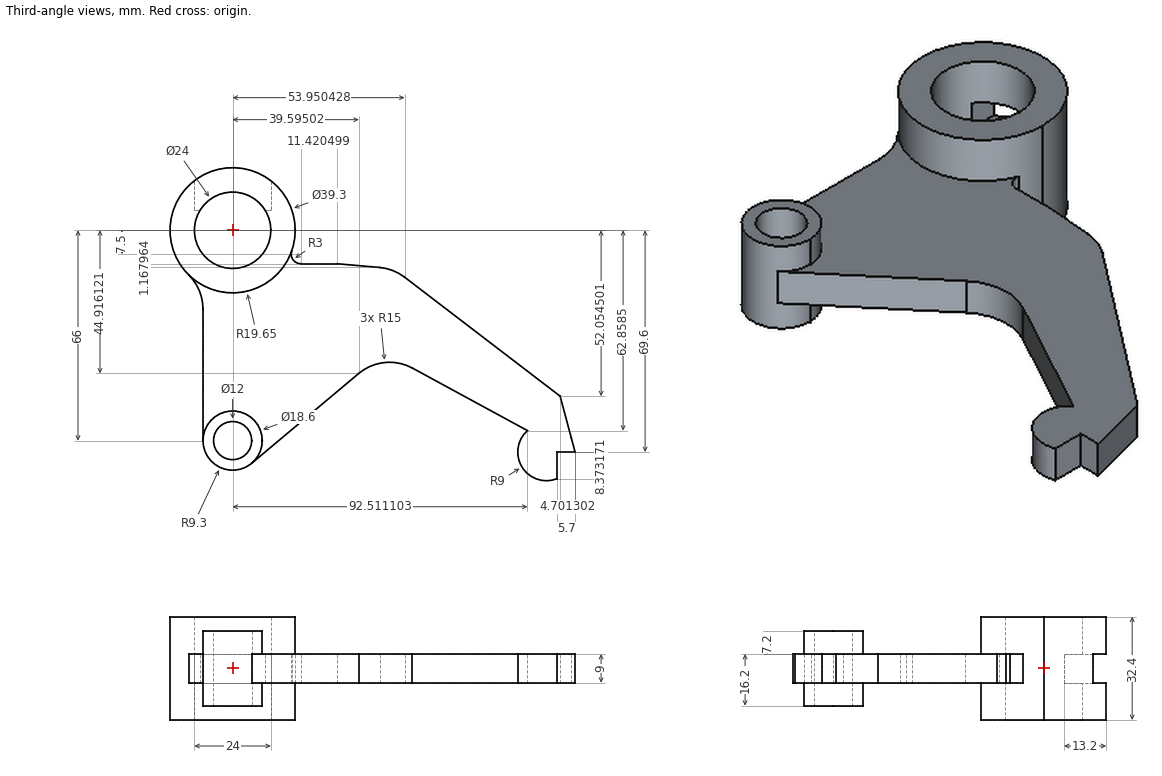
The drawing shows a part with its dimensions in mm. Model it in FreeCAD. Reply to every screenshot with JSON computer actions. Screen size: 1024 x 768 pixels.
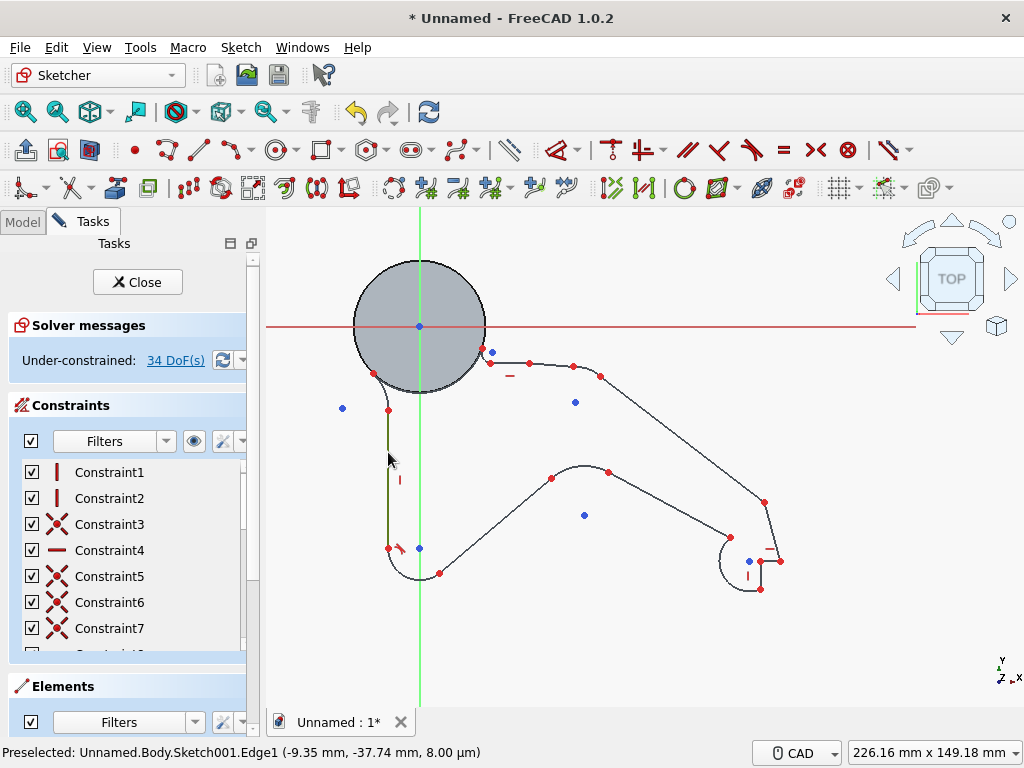
{"action": "left_click", "coordinate": [387, 399]}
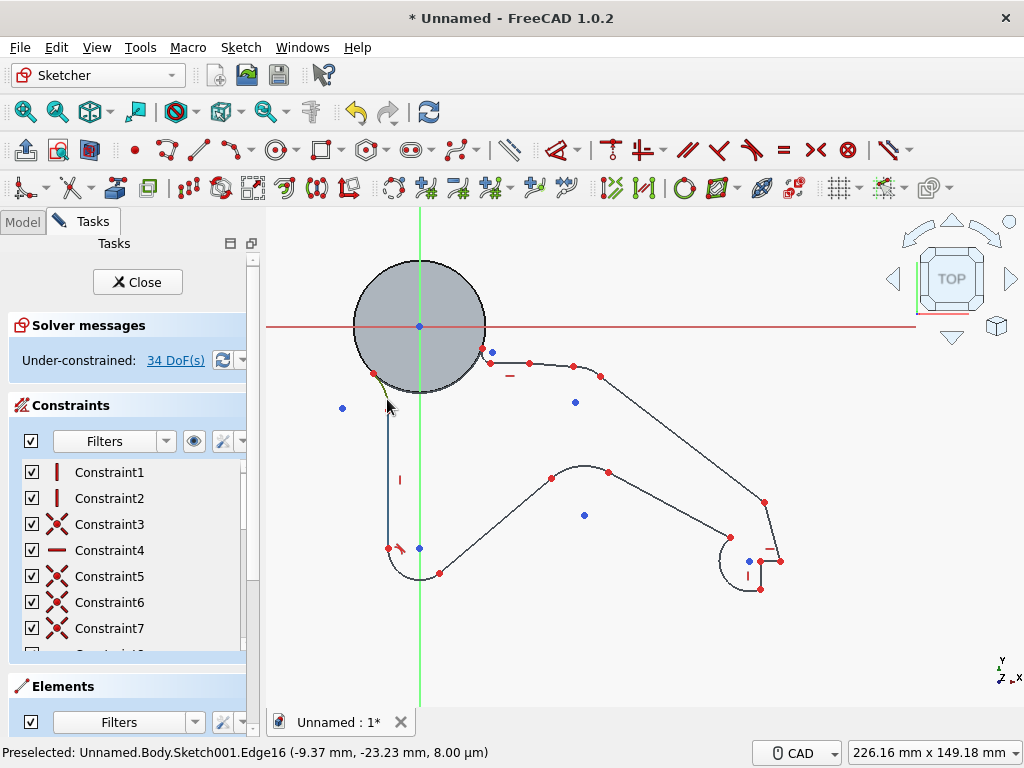
{"action": "key", "text": "t"}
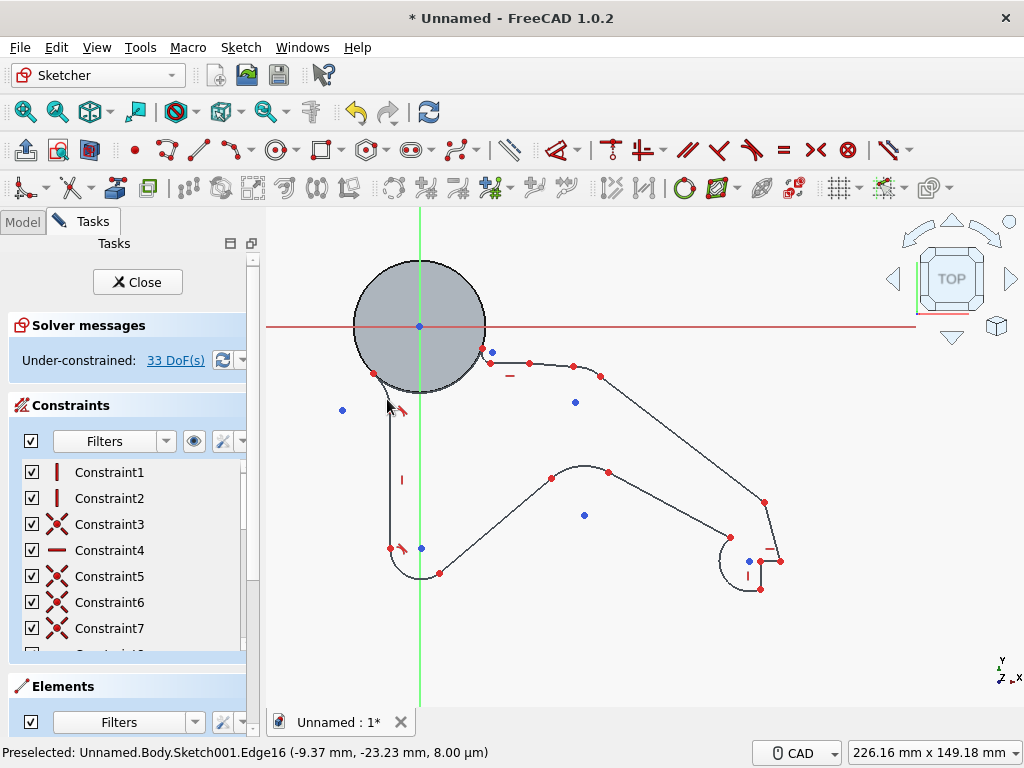
{"action": "left_click", "coordinate": [473, 545]}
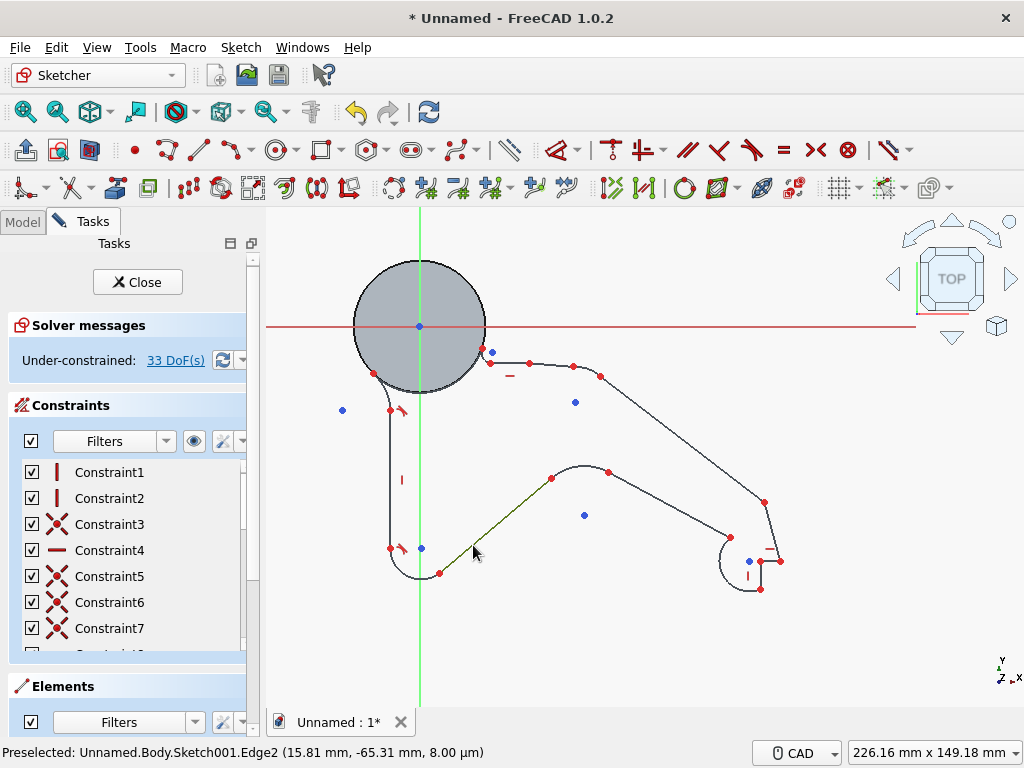
{"action": "left_click", "coordinate": [397, 567]}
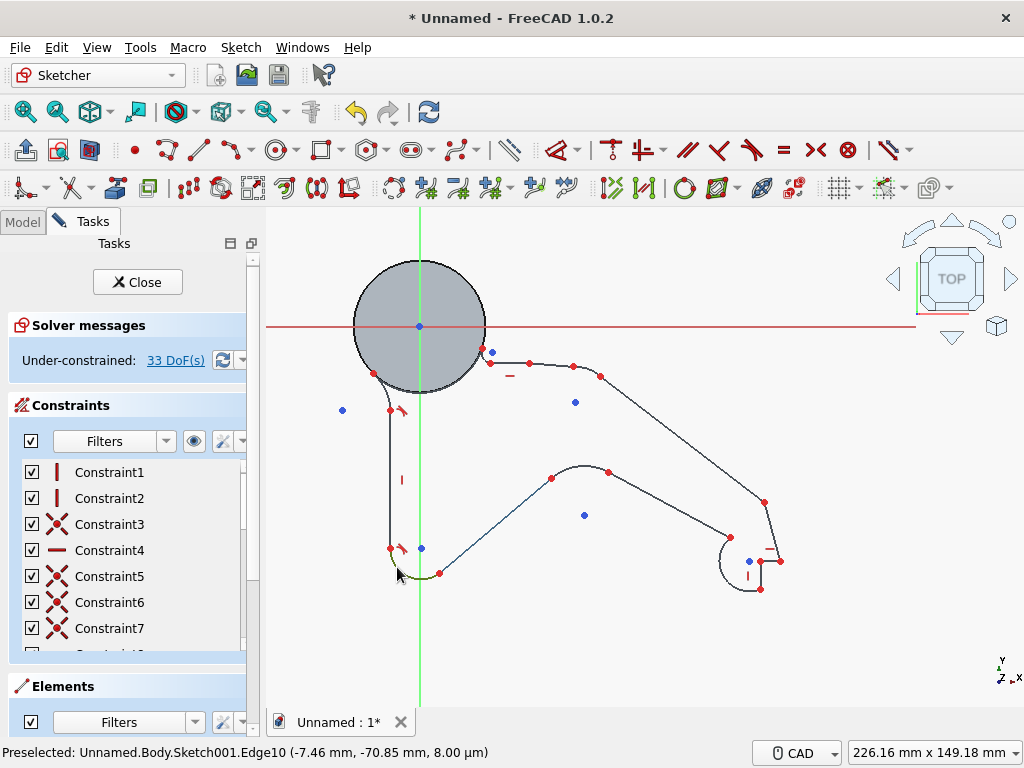
{"action": "key", "text": "t"}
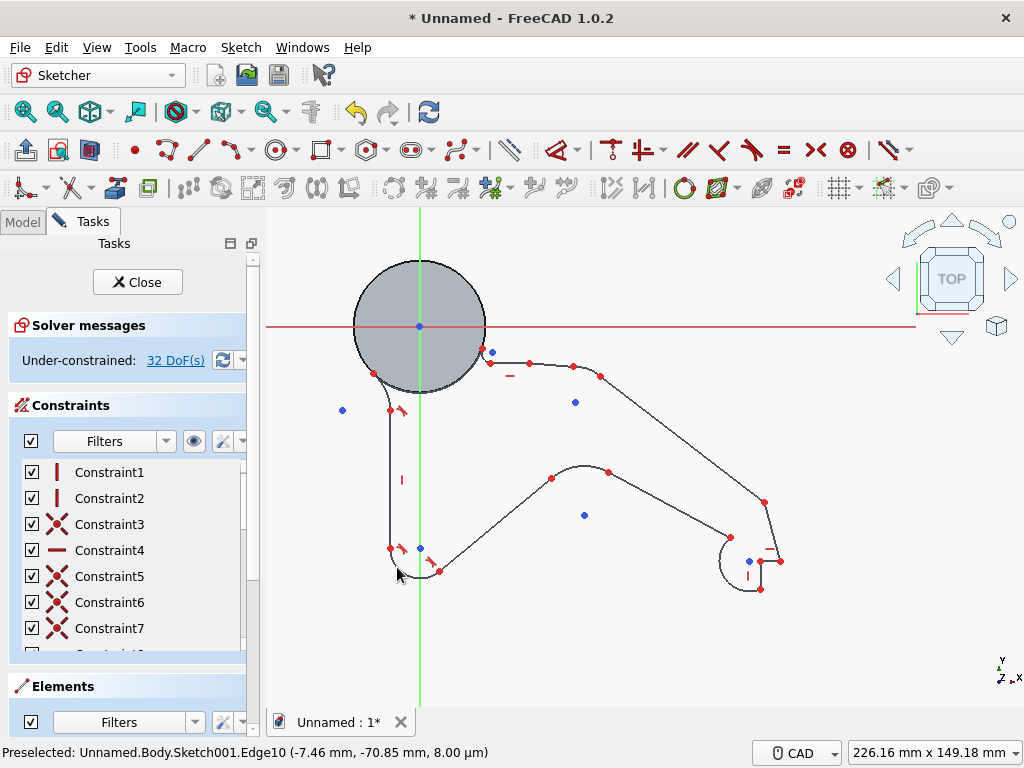
{"action": "left_click", "coordinate": [473, 543]}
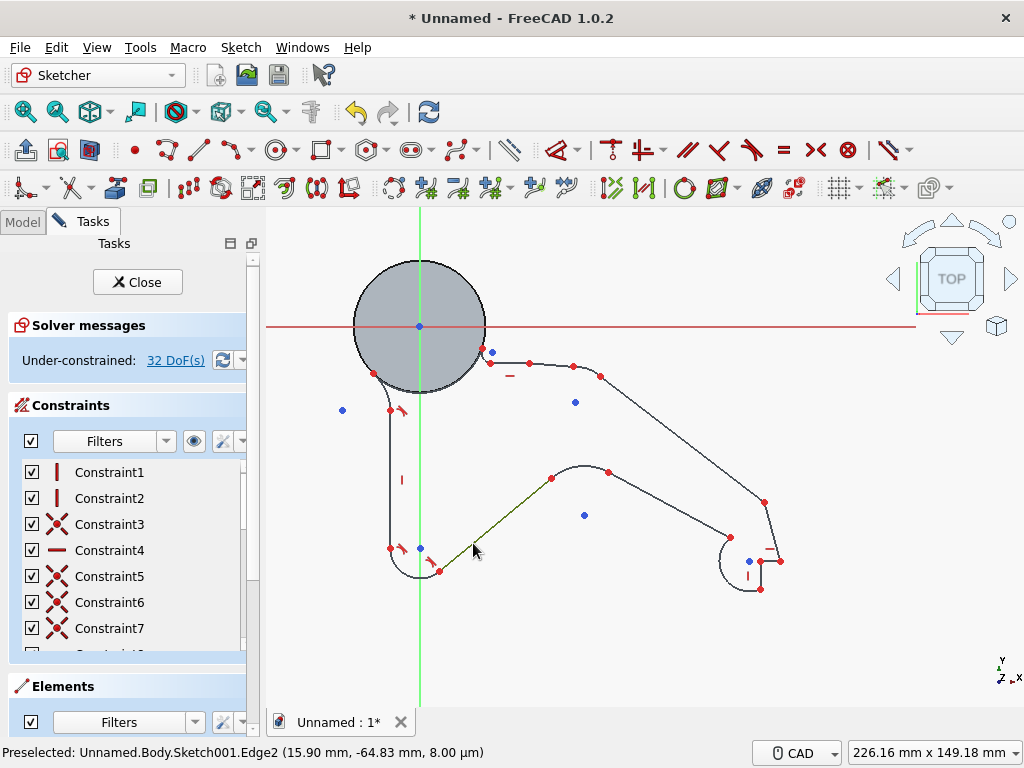
{"action": "left_click", "coordinate": [591, 466]}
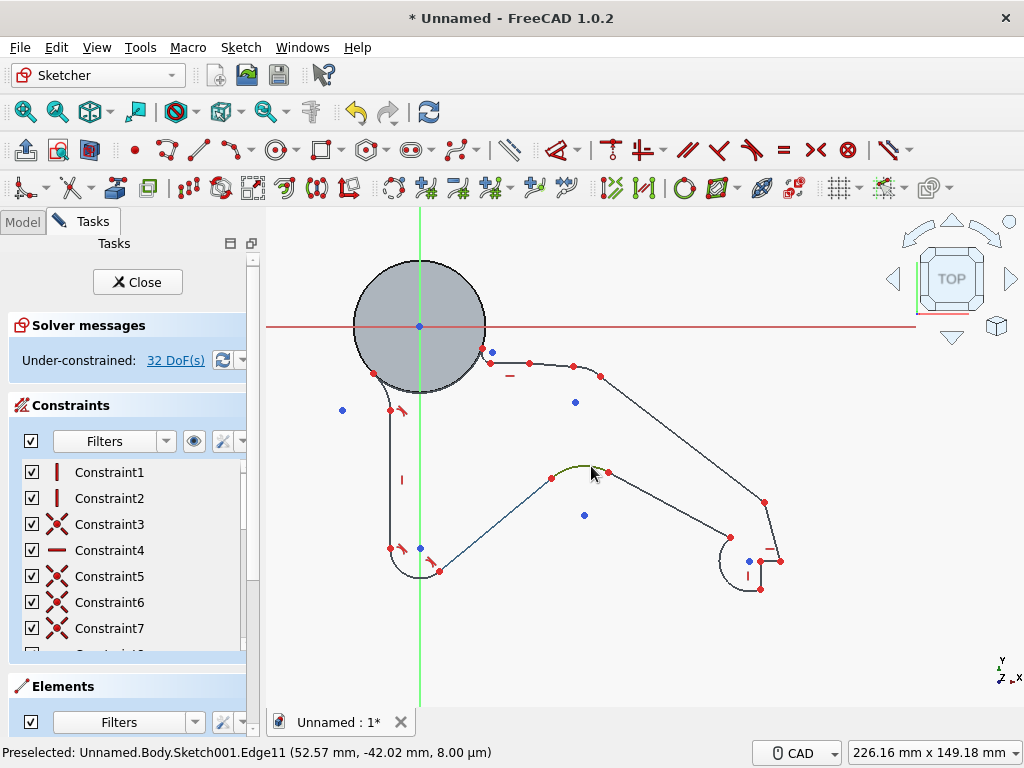
{"action": "key", "text": "t"}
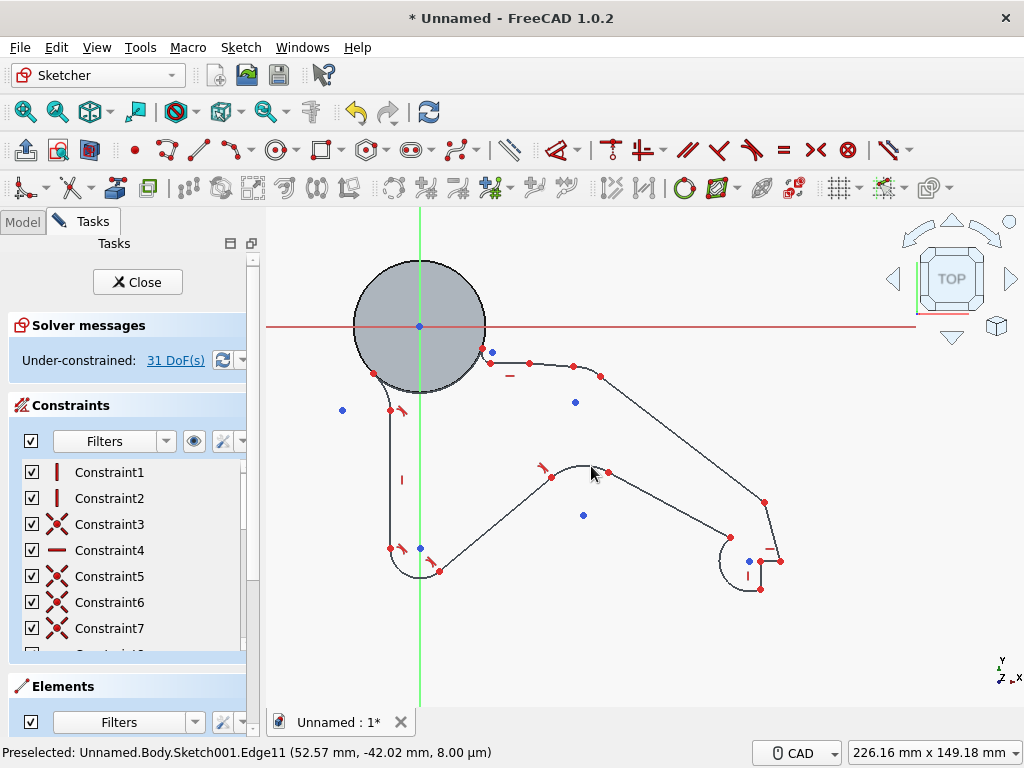
{"action": "left_click", "coordinate": [645, 492]}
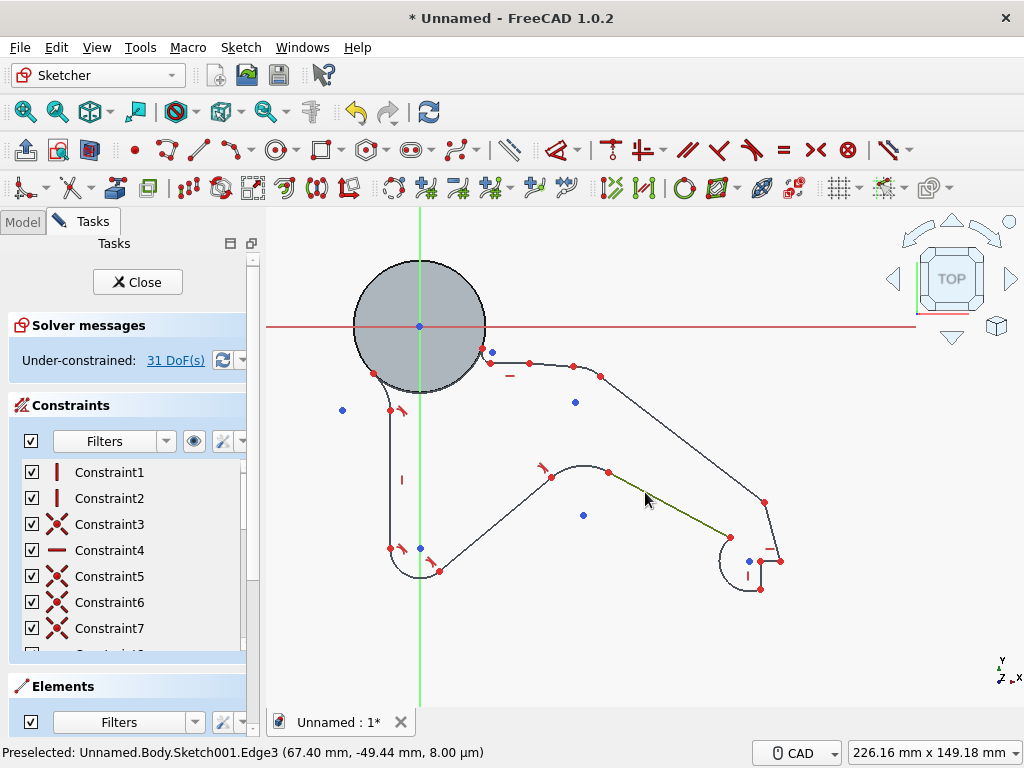
{"action": "left_click", "coordinate": [591, 466]}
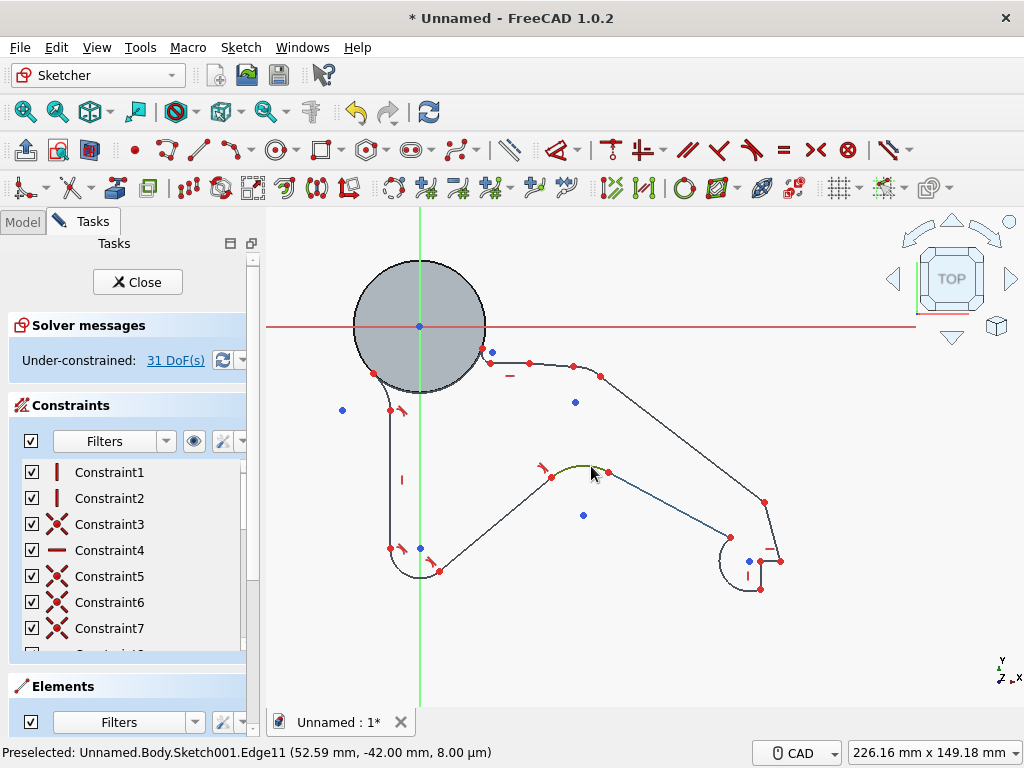
{"action": "key", "text": "t"}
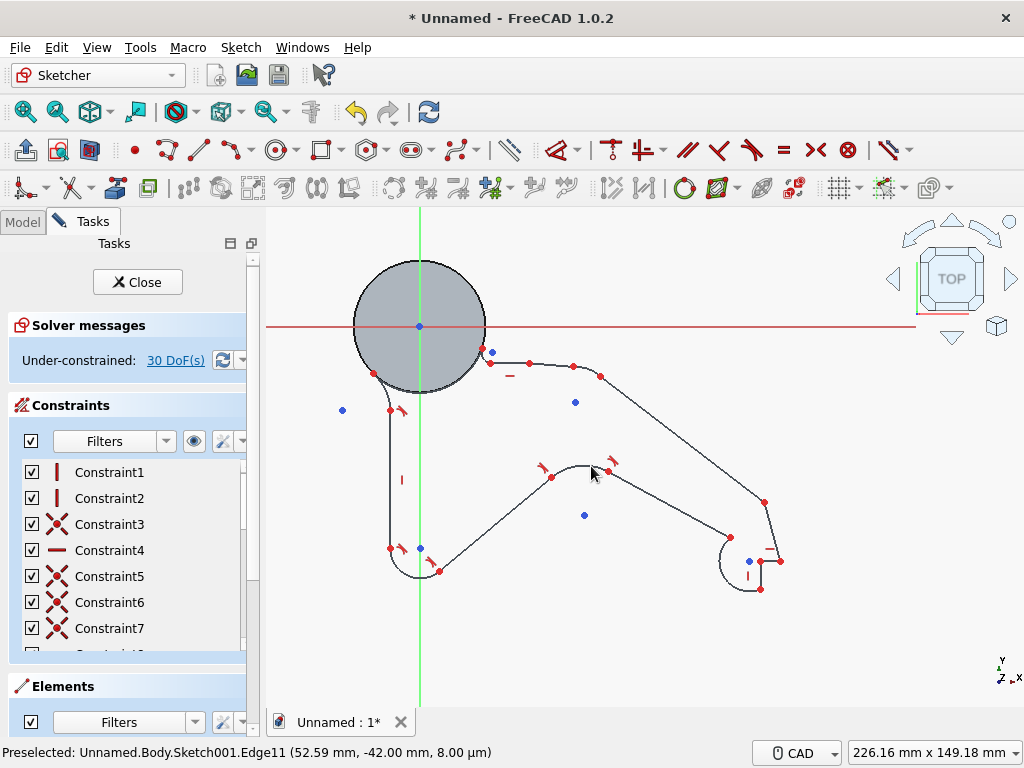
{"action": "left_click", "coordinate": [715, 465]}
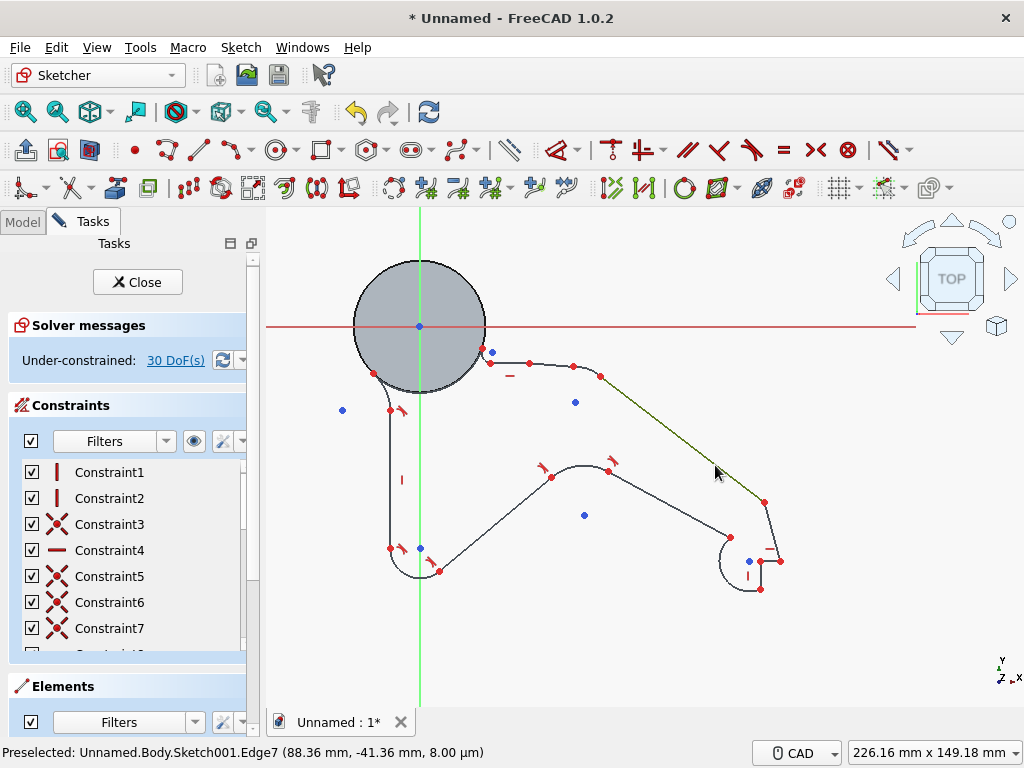
{"action": "left_click", "coordinate": [588, 369]}